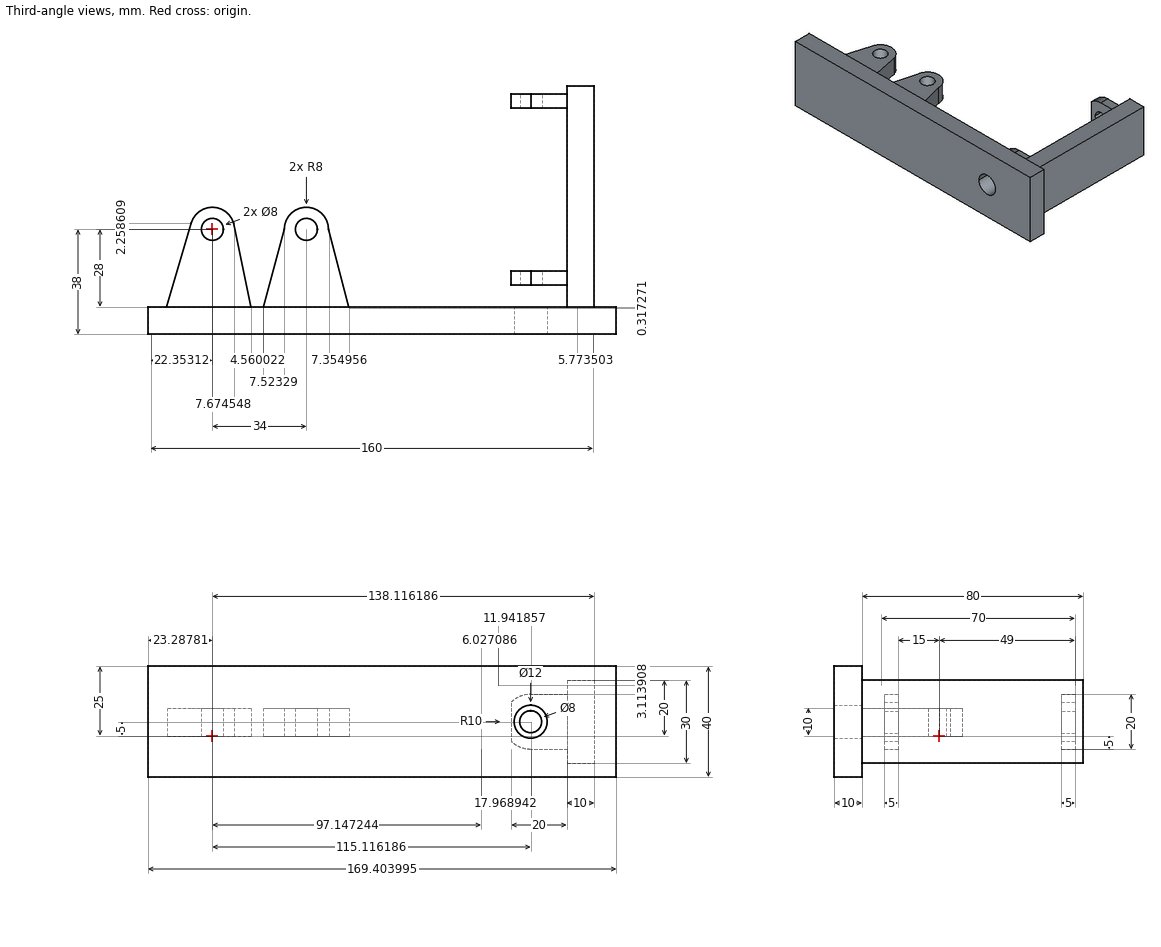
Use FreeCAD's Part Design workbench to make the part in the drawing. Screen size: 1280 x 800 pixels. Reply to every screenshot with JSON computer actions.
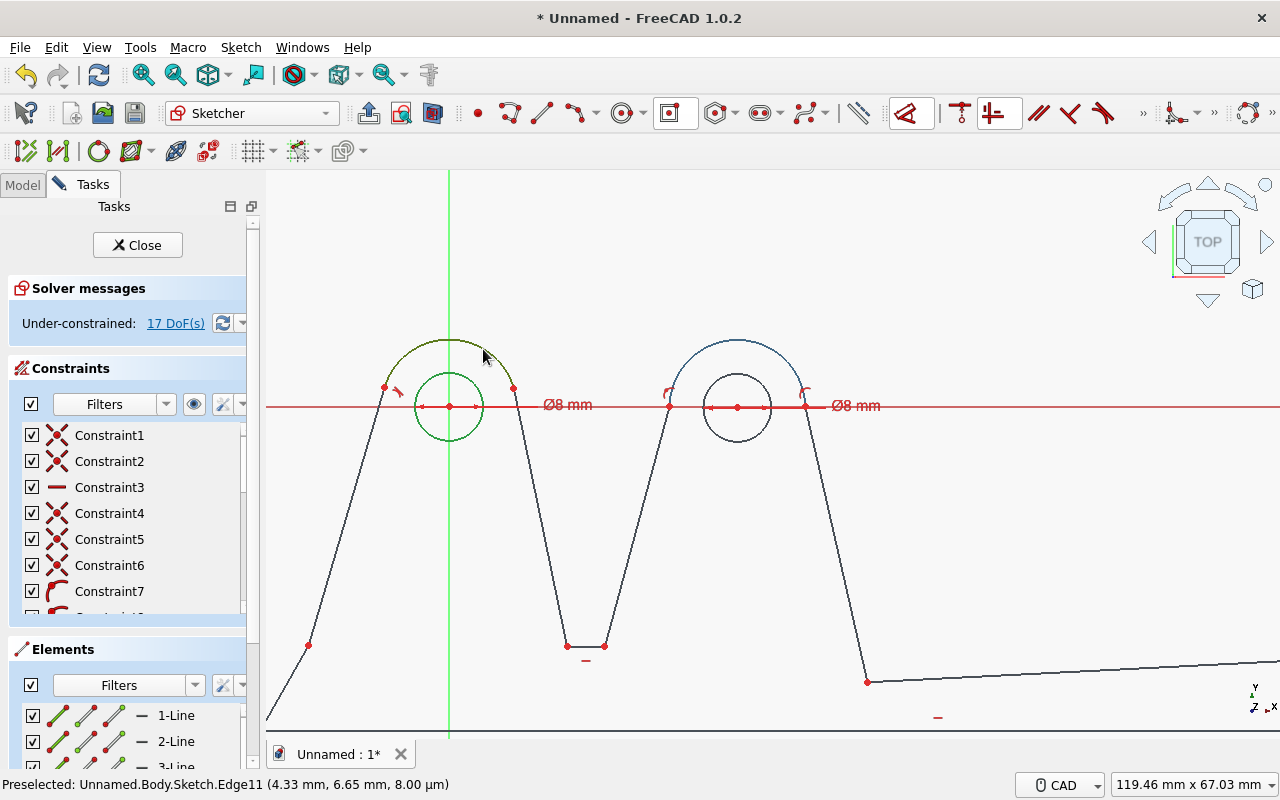
{"action": "key", "text": "e"}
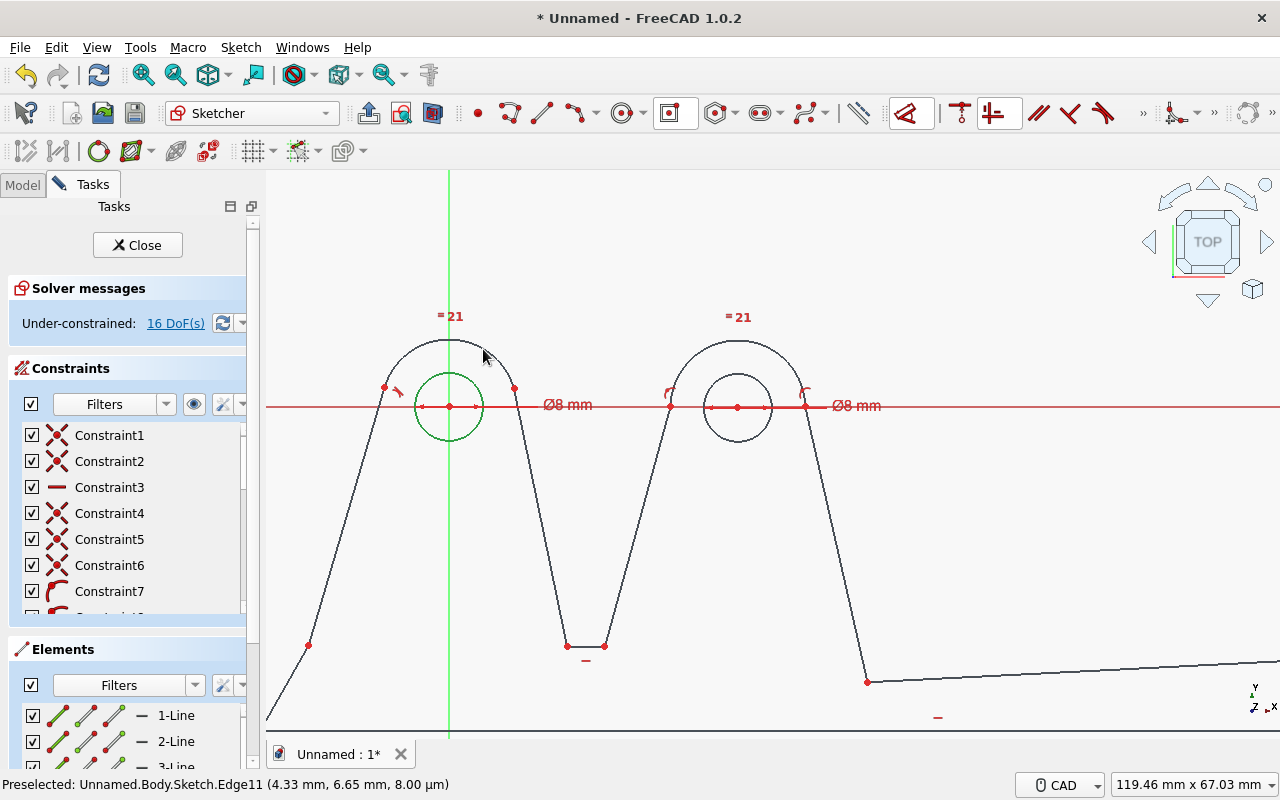
{"action": "left_click", "coordinate": [738, 408]}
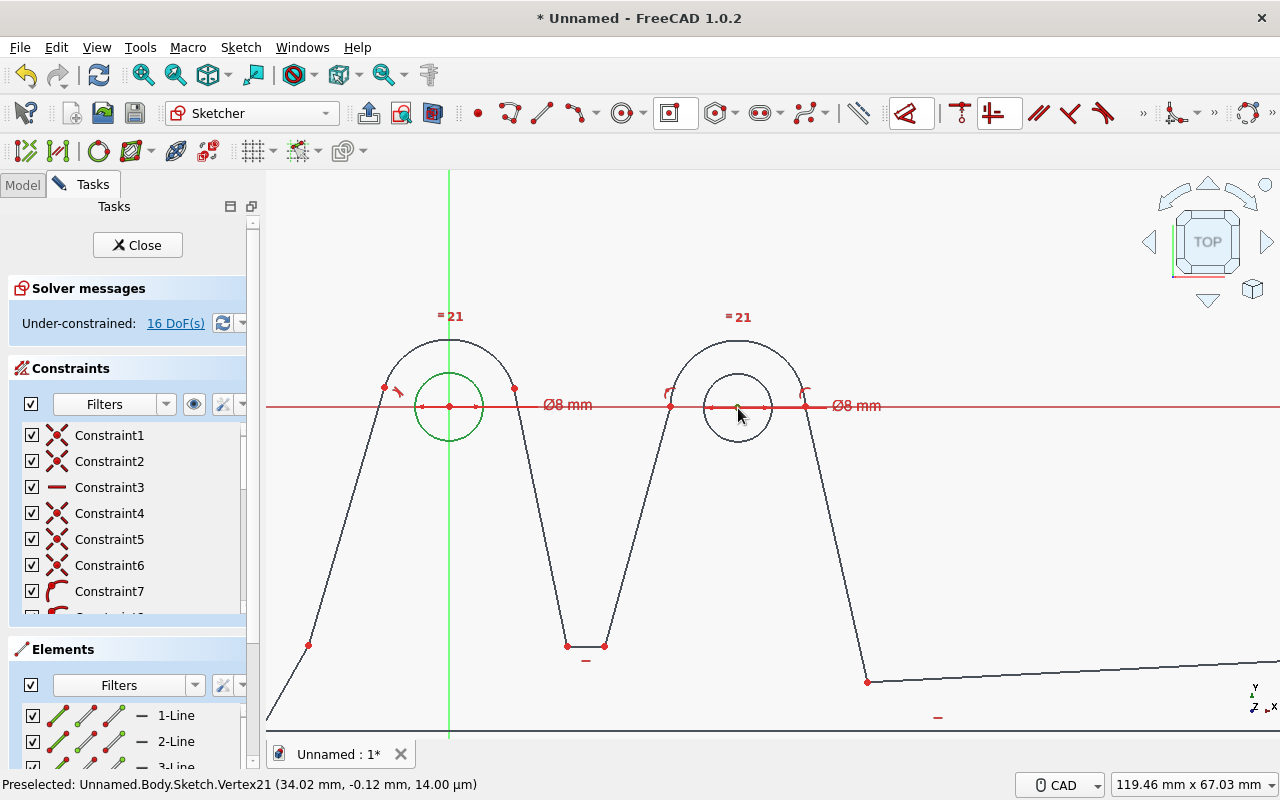
{"action": "left_click", "coordinate": [939, 407]}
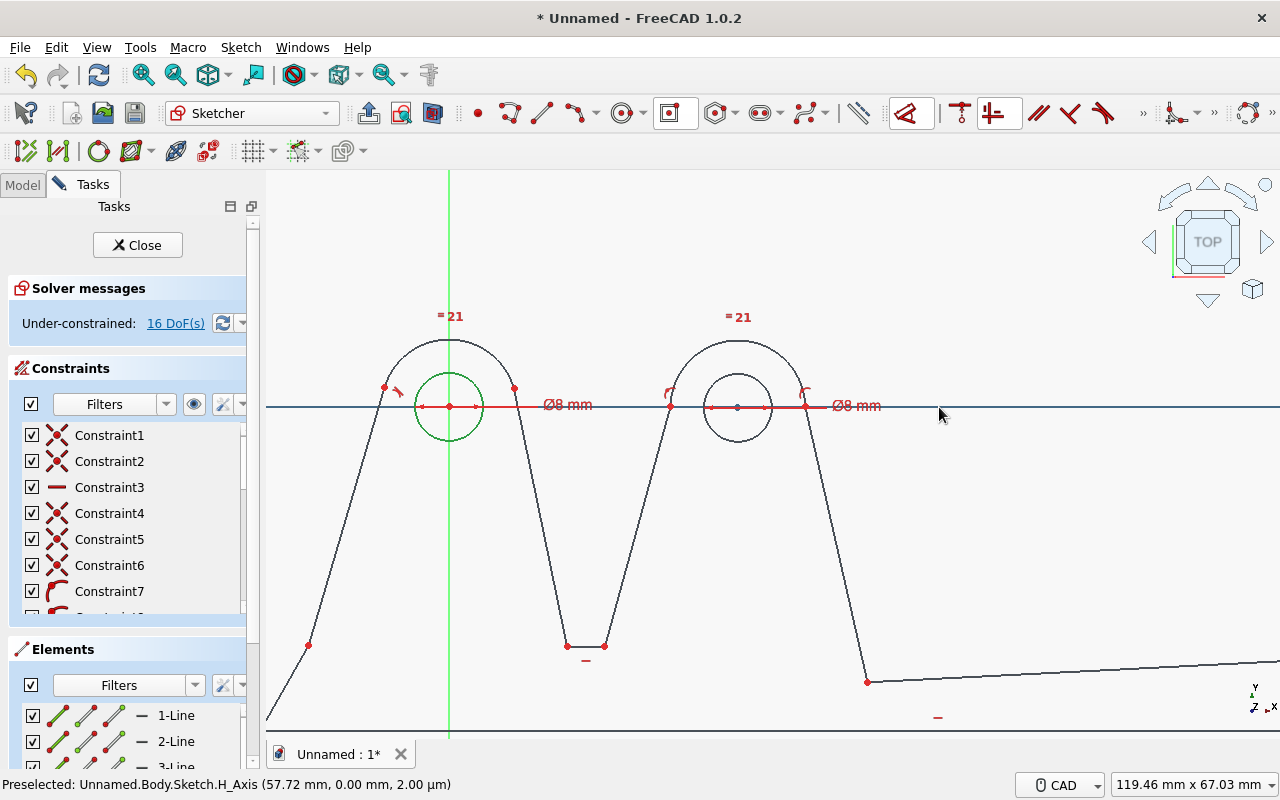
{"action": "left_click", "coordinate": [960, 114]}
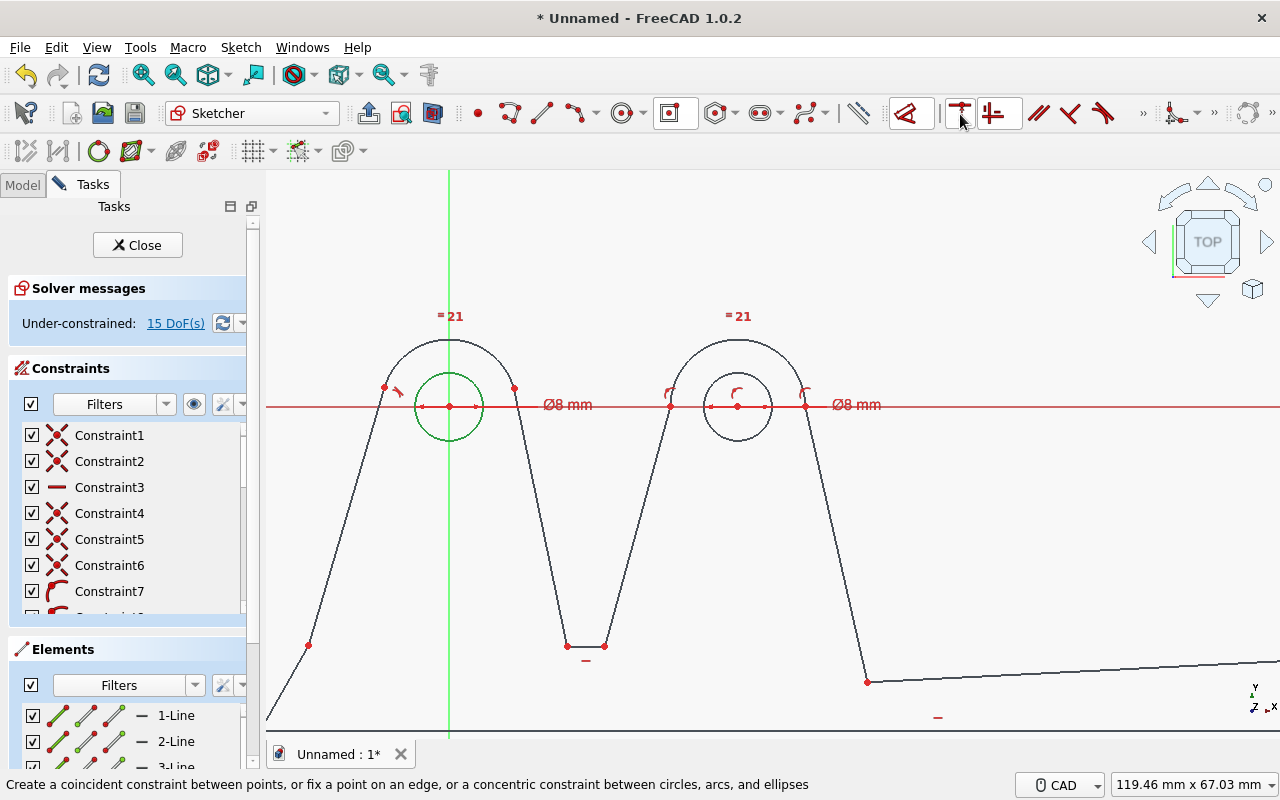
{"action": "left_click", "coordinate": [906, 114]}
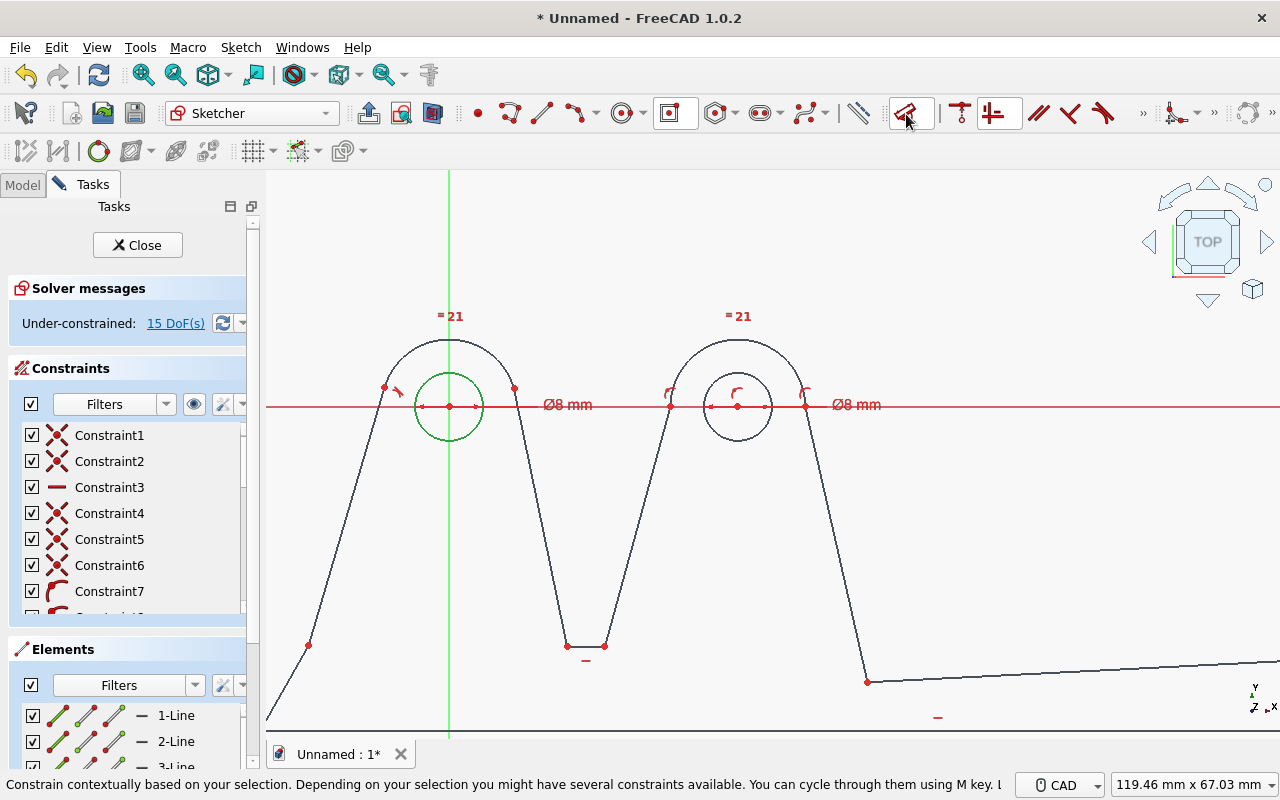
{"action": "left_click", "coordinate": [777, 352]}
{"action": "left_click", "coordinate": [796, 326]}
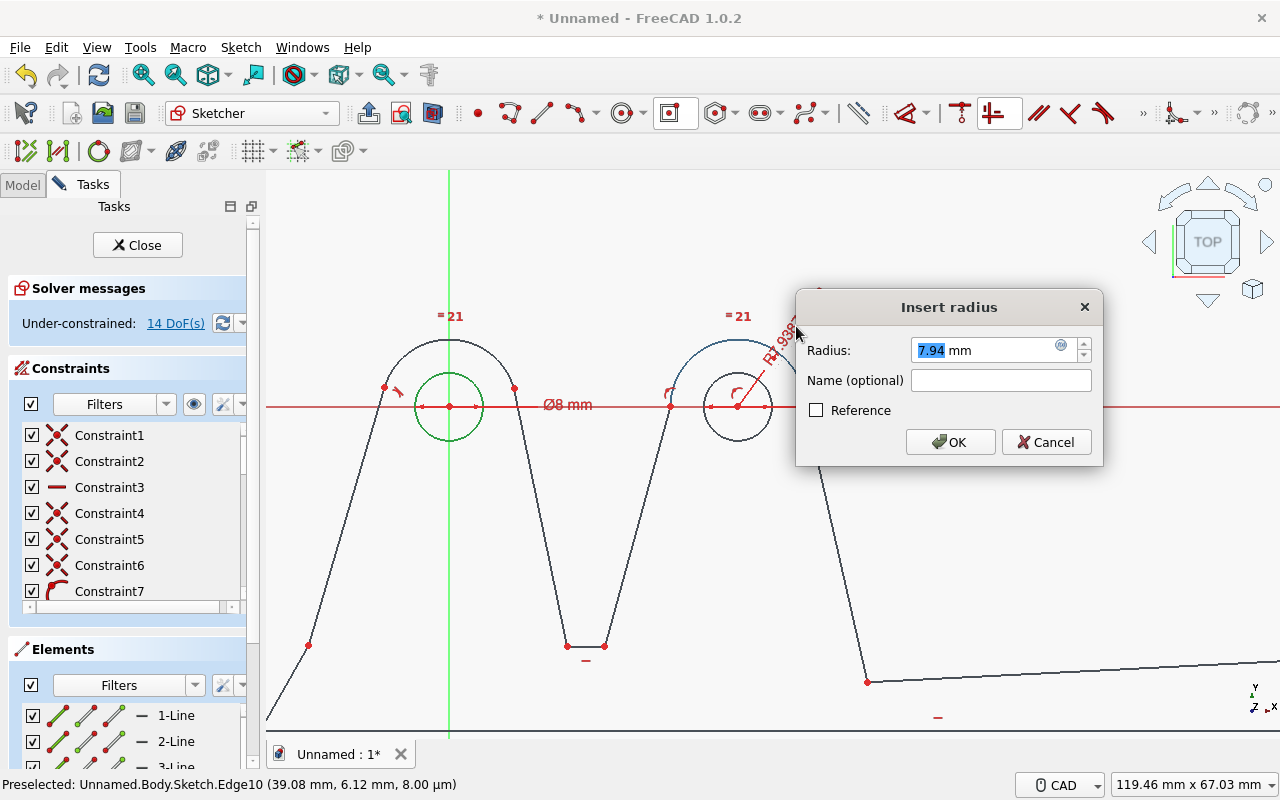
{"action": "type", "text": "8"}
{"action": "key", "text": "Return"}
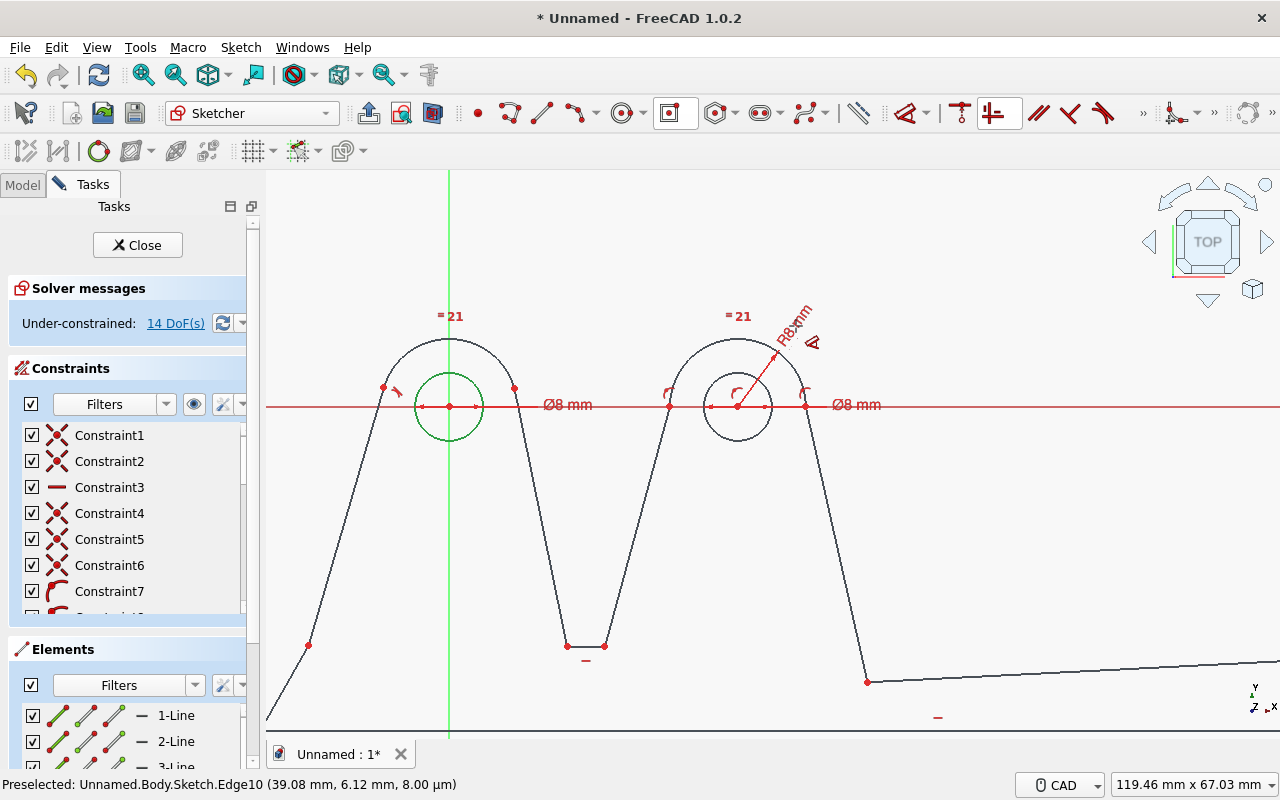
{"action": "left_click", "coordinate": [738, 407]}
{"action": "left_click", "coordinate": [593, 373]}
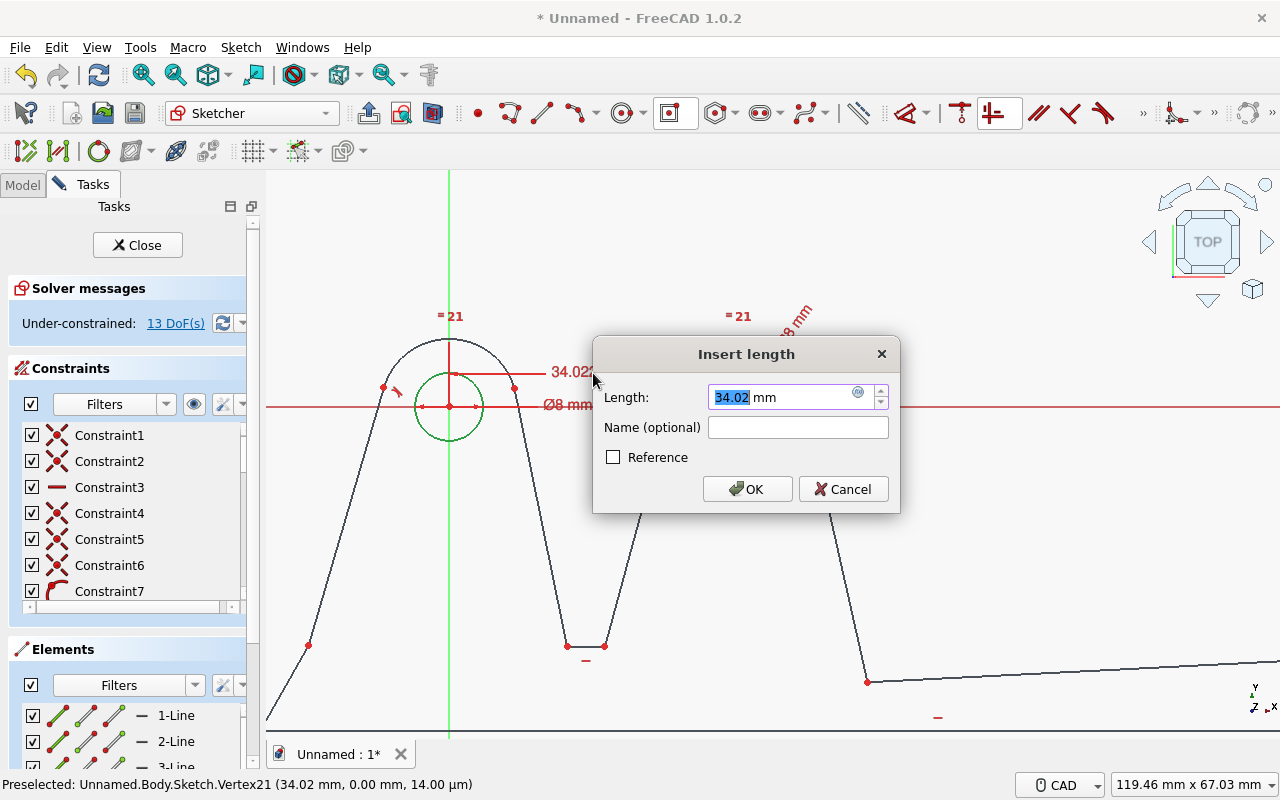
{"action": "type", "text": "34"}
{"action": "key", "text": "Return"}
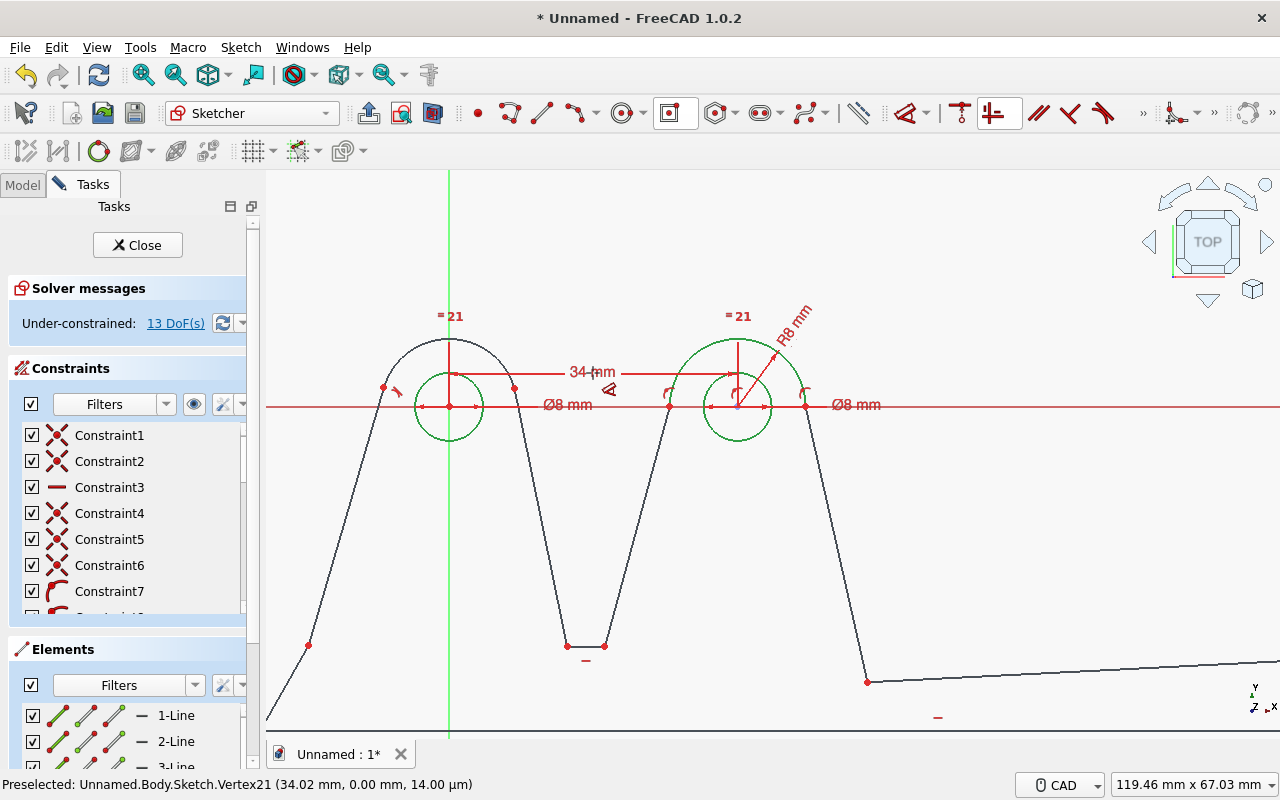
{"action": "scroll", "coordinate": [514, 389], "scroll_direction": "down", "scroll_amount": 4}